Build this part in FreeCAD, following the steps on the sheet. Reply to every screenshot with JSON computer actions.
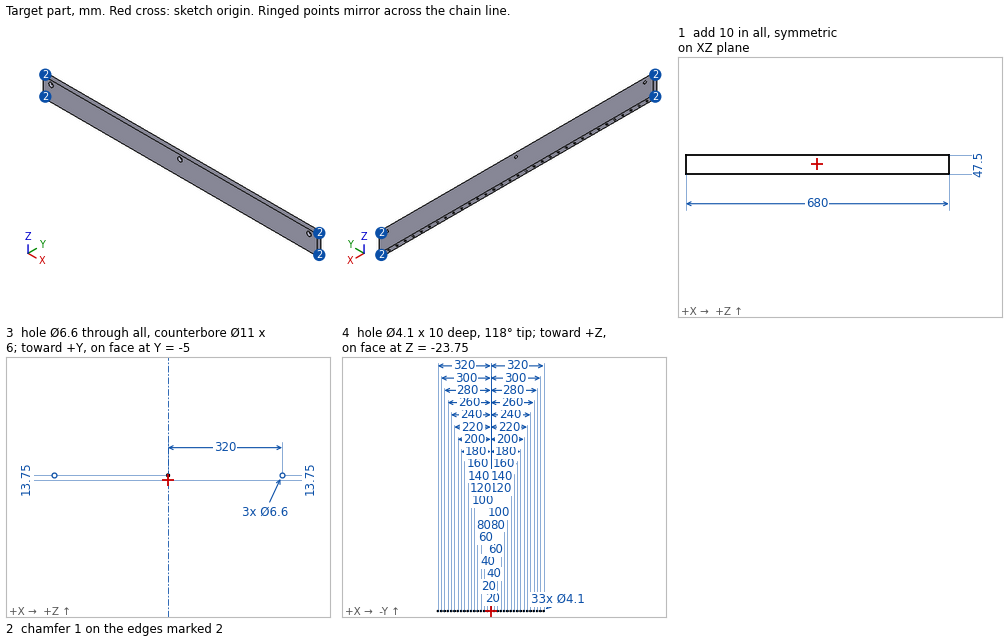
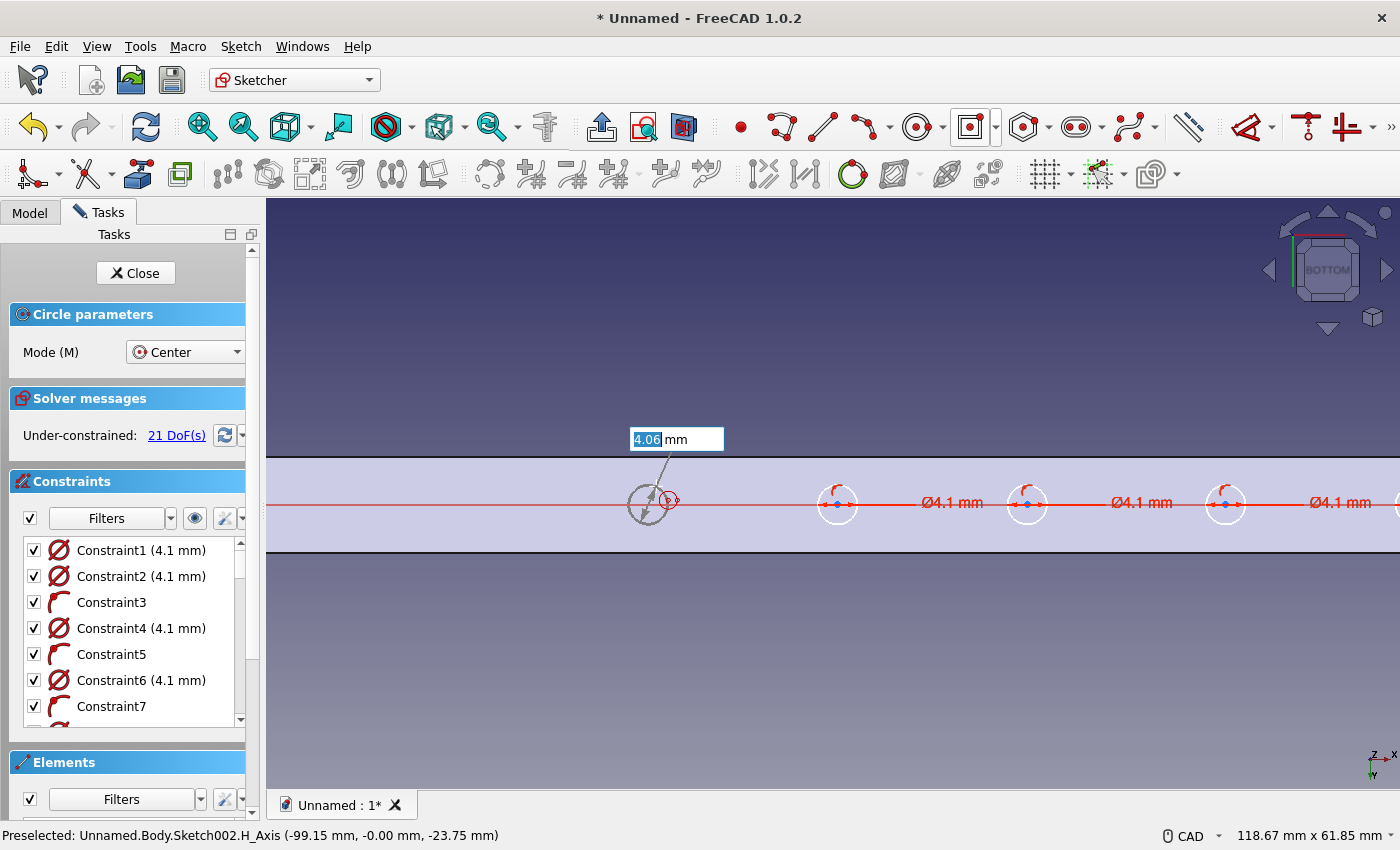
{"action": "type", "text": "4.1"}
{"action": "key", "text": "Return"}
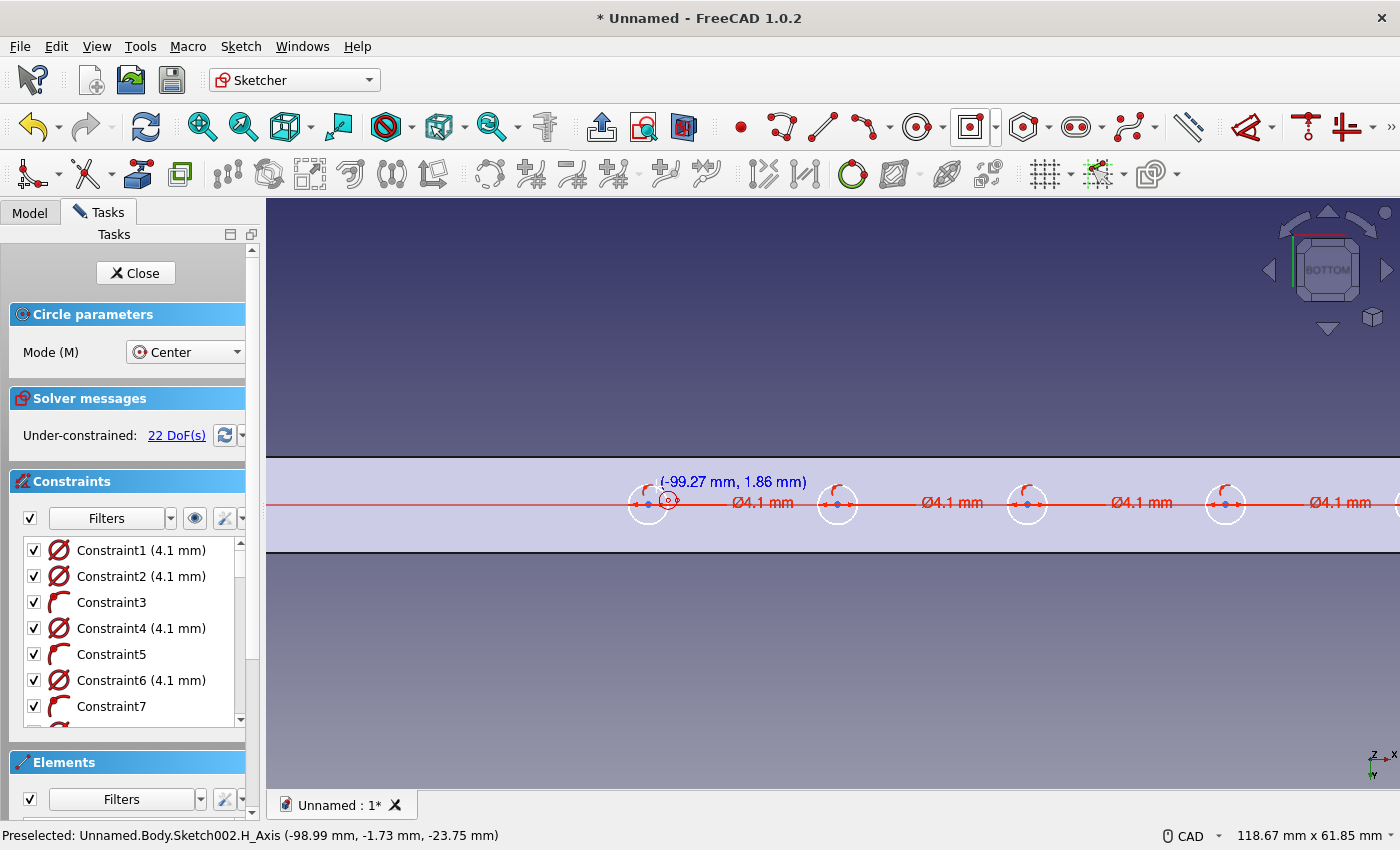
{"action": "scroll", "coordinate": [660, 492], "scroll_direction": "down", "scroll_amount": 11}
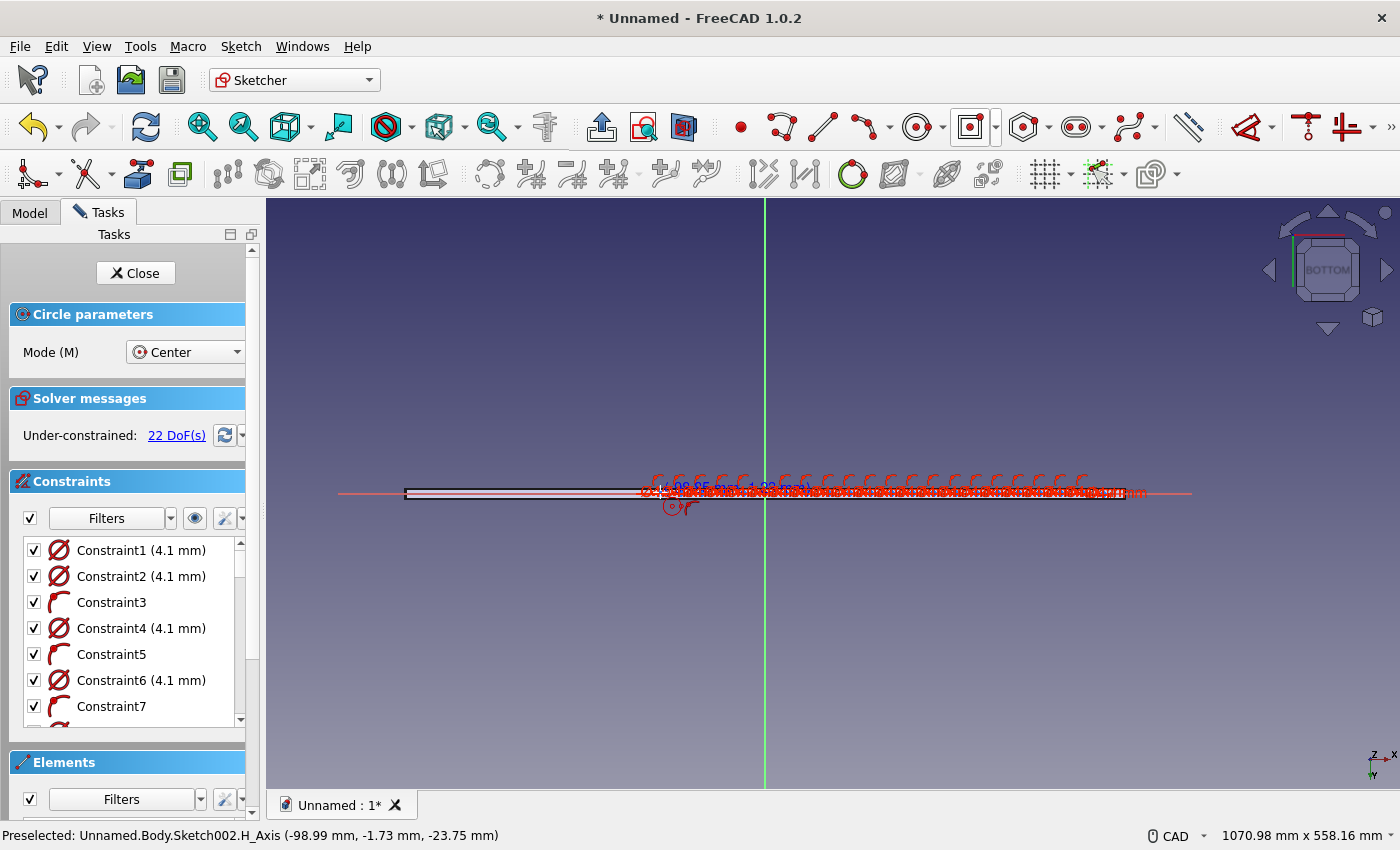
{"action": "left_click", "coordinate": [638, 494]}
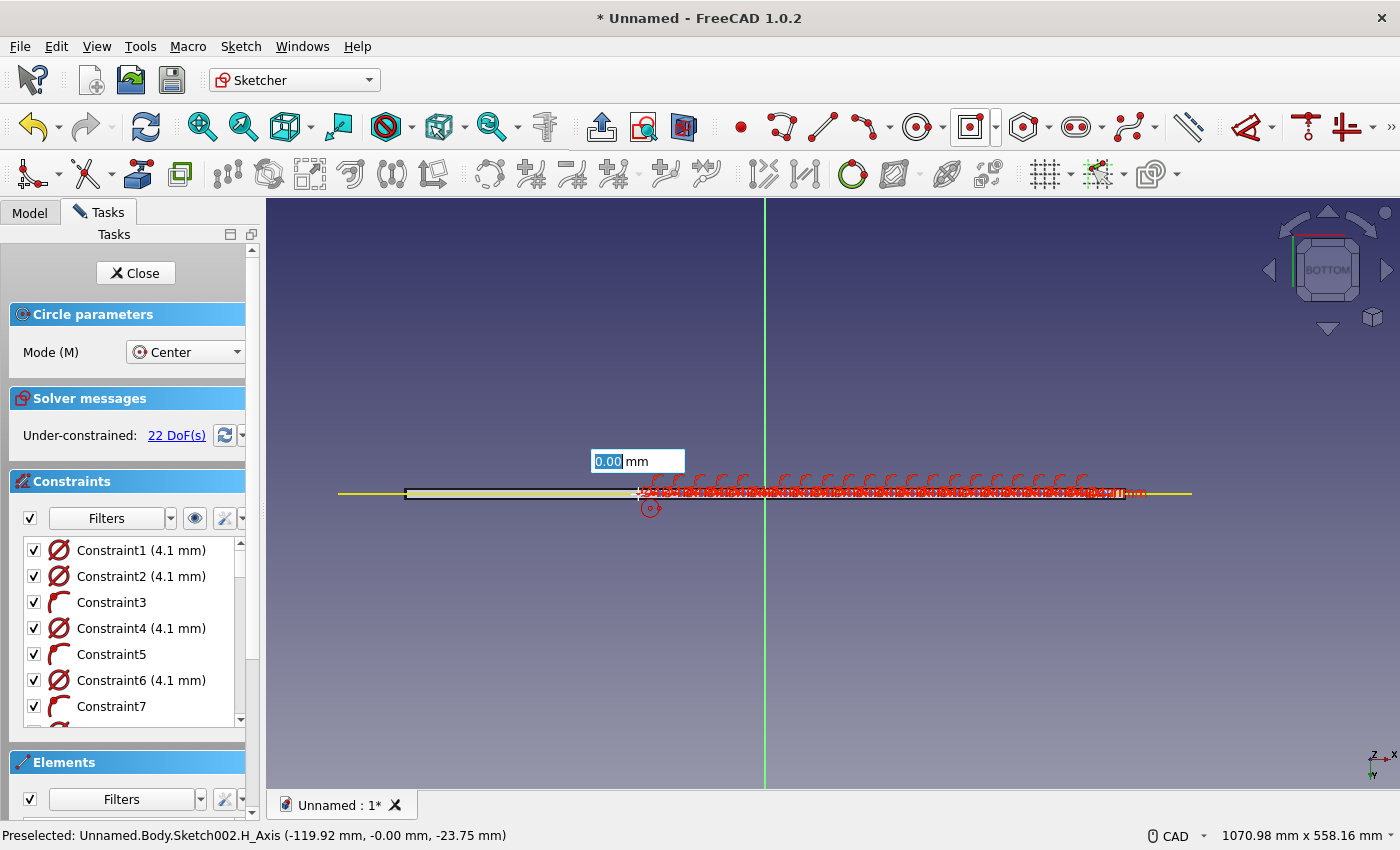
{"action": "scroll", "coordinate": [639, 492], "scroll_direction": "up", "scroll_amount": 11}
{"action": "mouse_move", "coordinate": [633, 486]}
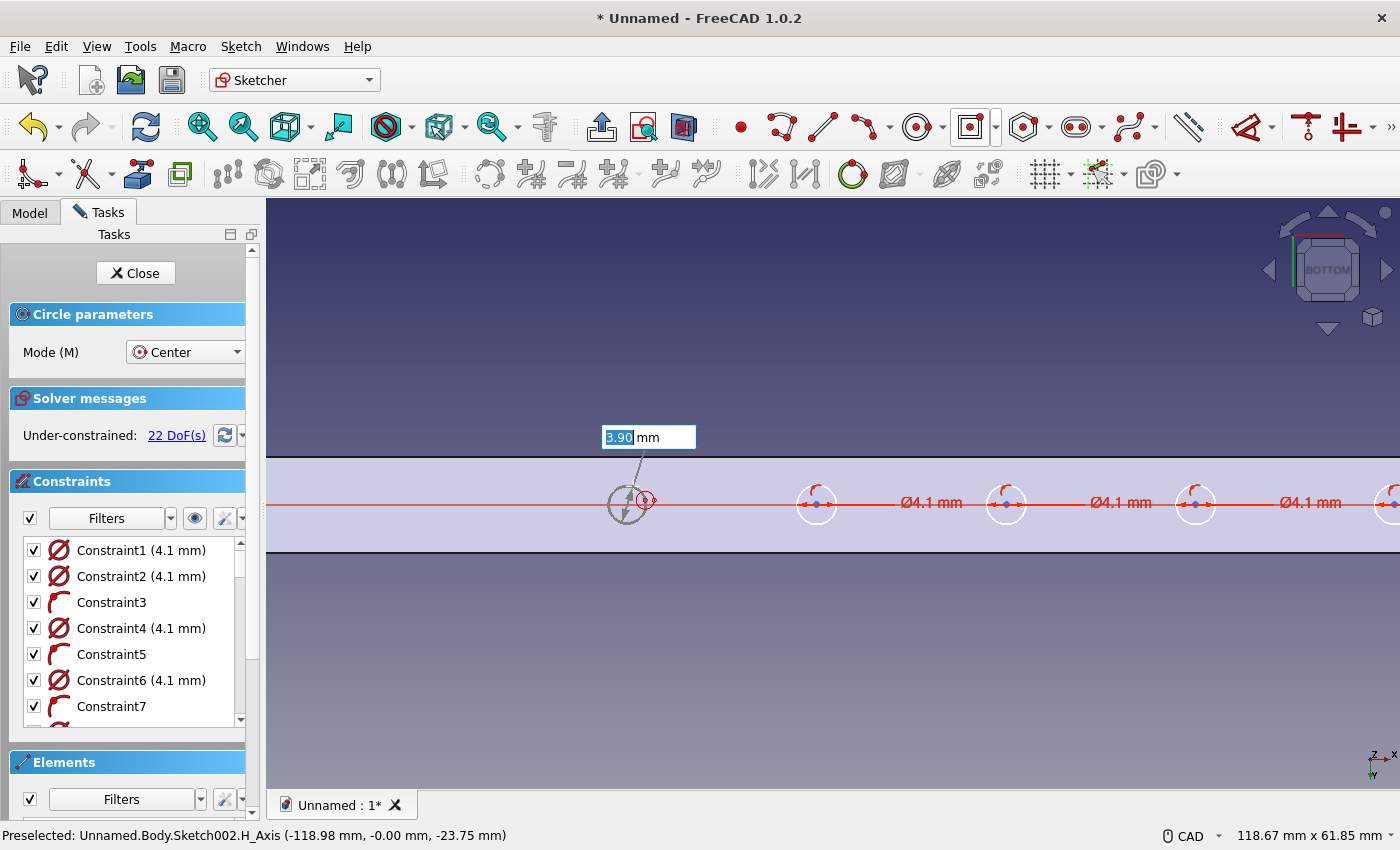
{"action": "type", "text": "4.1"}
{"action": "key", "text": "Return"}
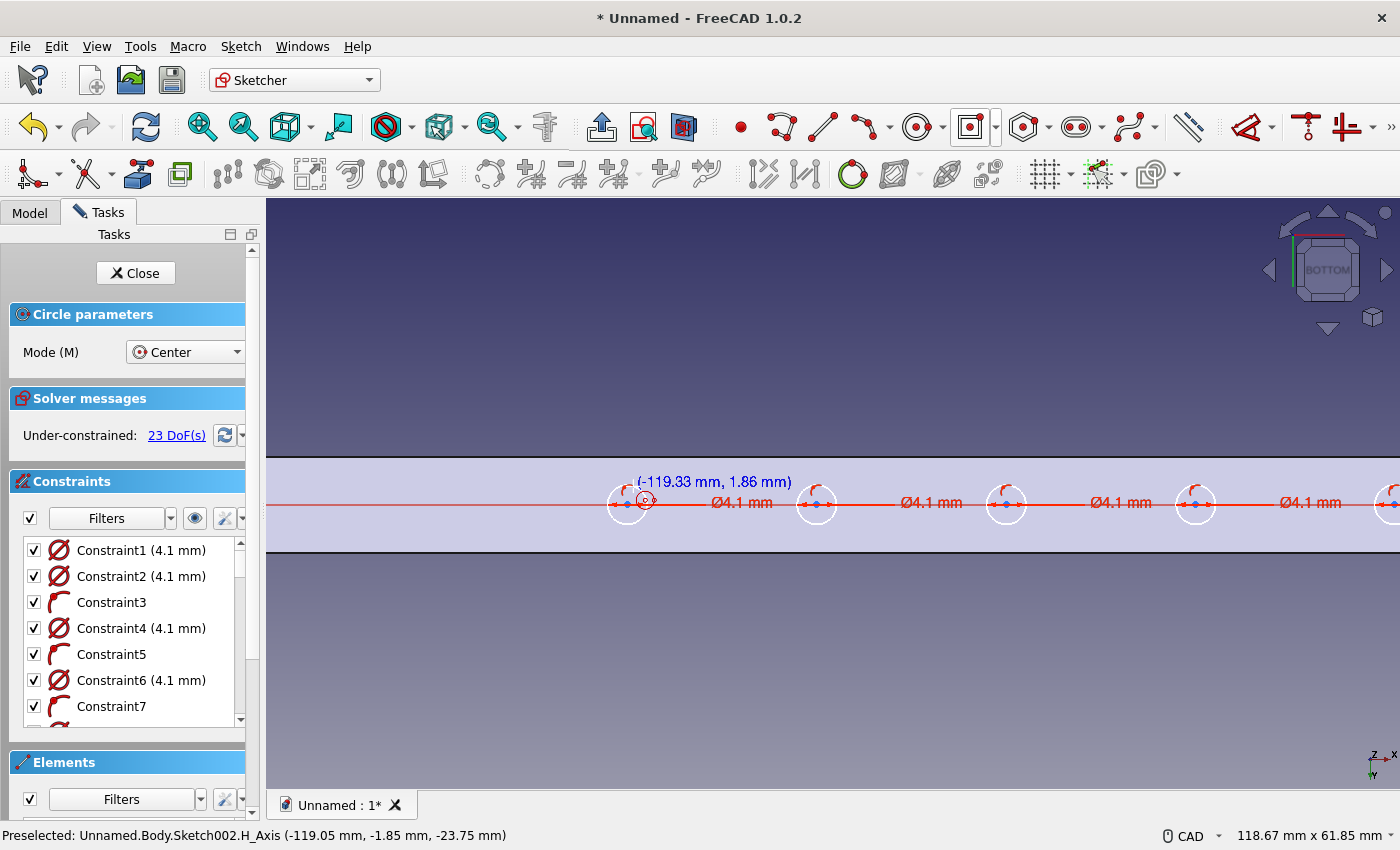
{"action": "scroll", "coordinate": [639, 492], "scroll_direction": "down", "scroll_amount": 11}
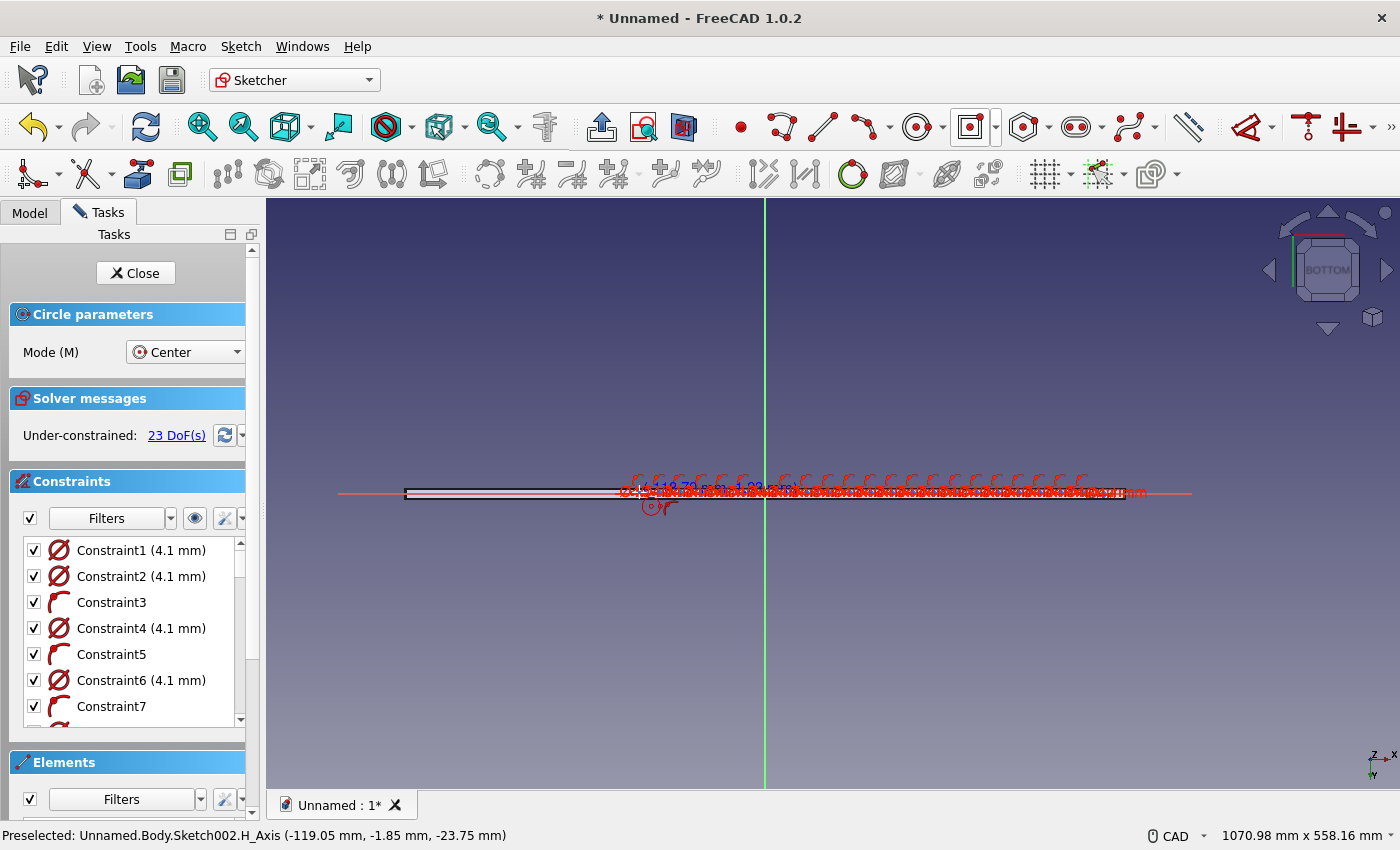
{"action": "left_click", "coordinate": [617, 494]}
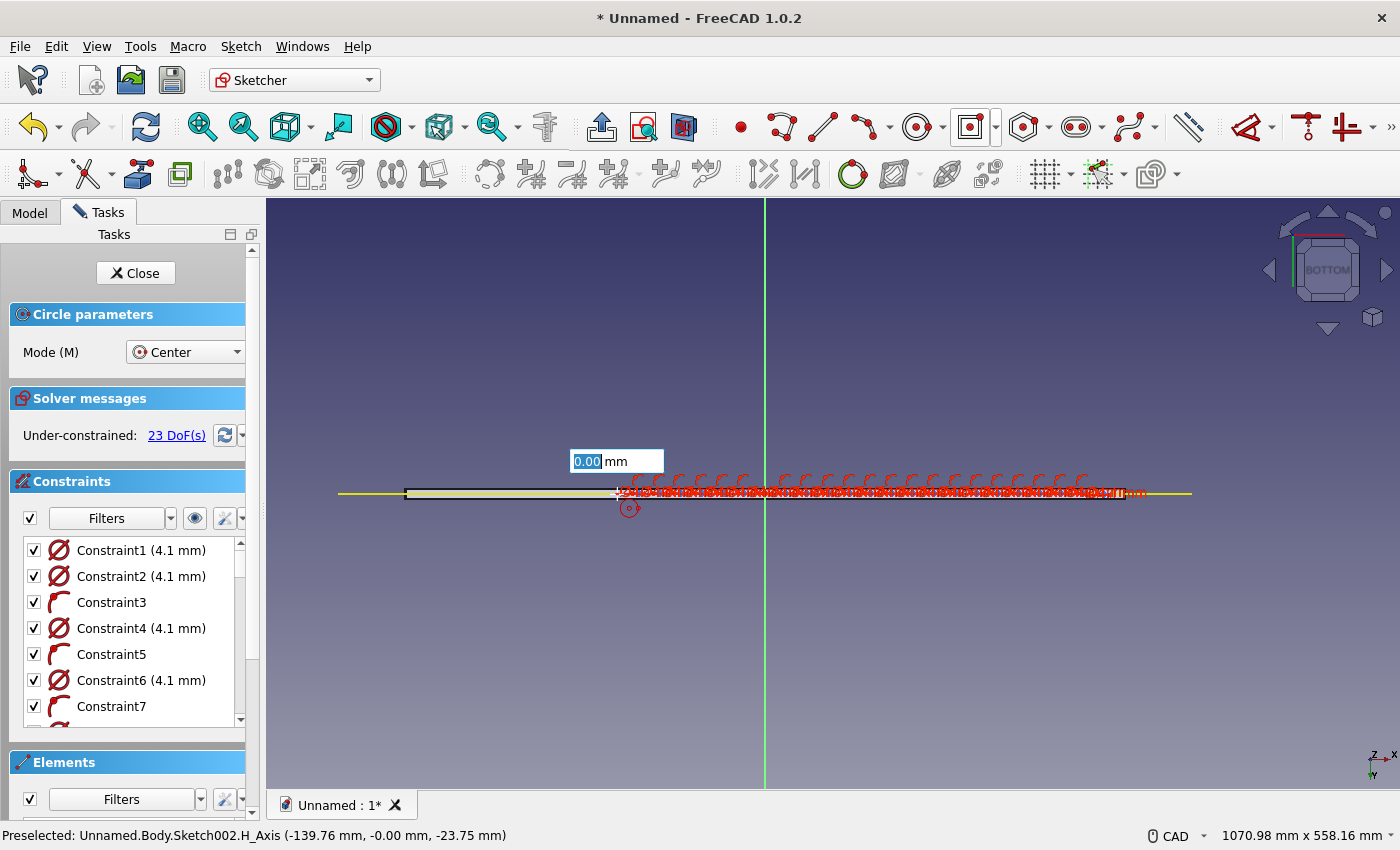
{"action": "scroll", "coordinate": [617, 492], "scroll_direction": "up", "scroll_amount": 11}
{"action": "mouse_move", "coordinate": [619, 486]}